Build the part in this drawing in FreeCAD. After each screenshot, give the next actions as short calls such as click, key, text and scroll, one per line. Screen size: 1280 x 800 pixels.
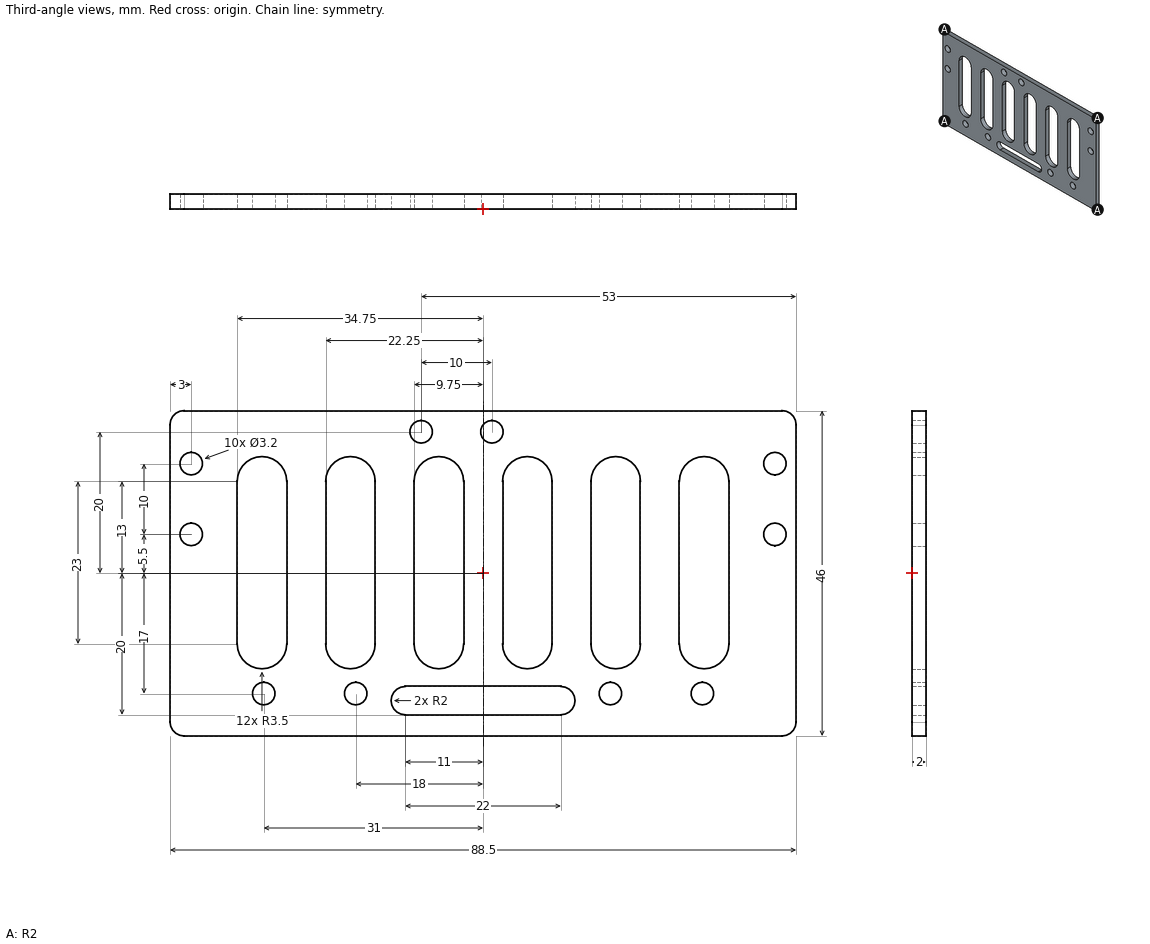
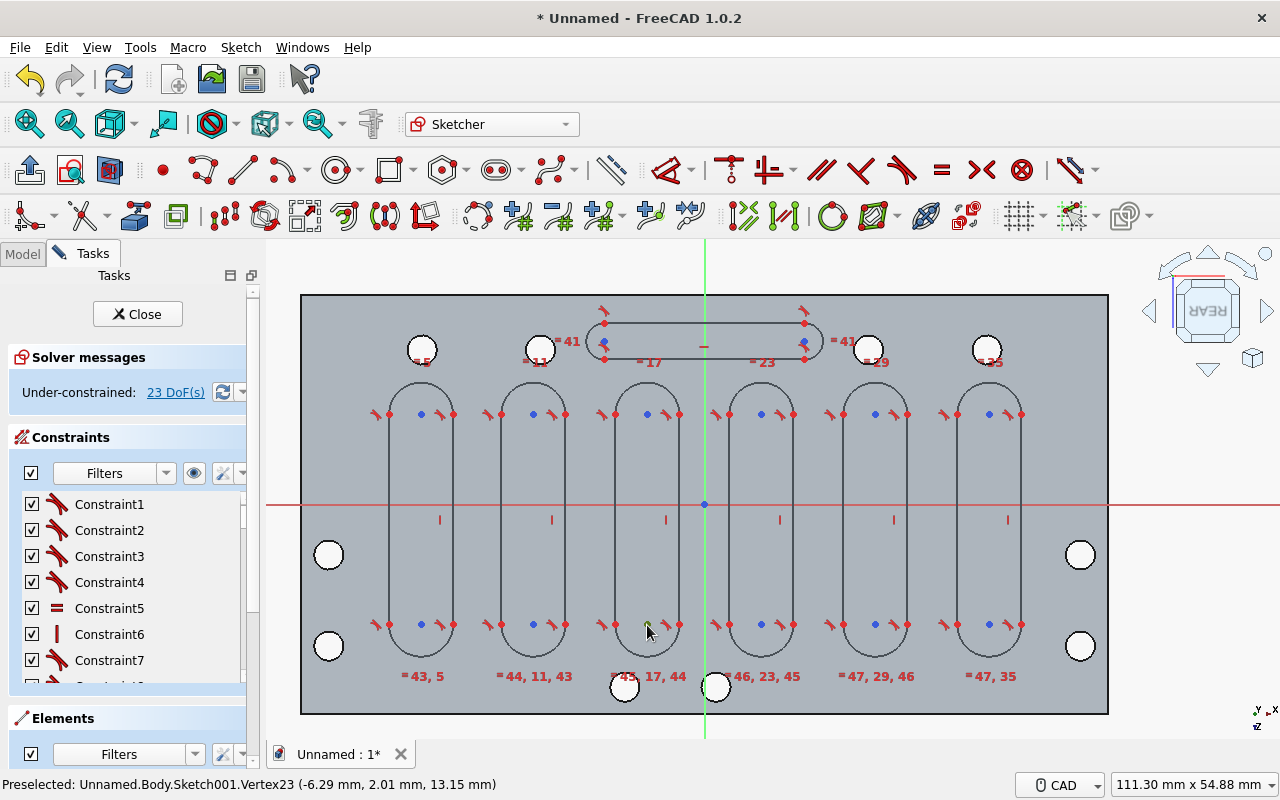
click(761, 625)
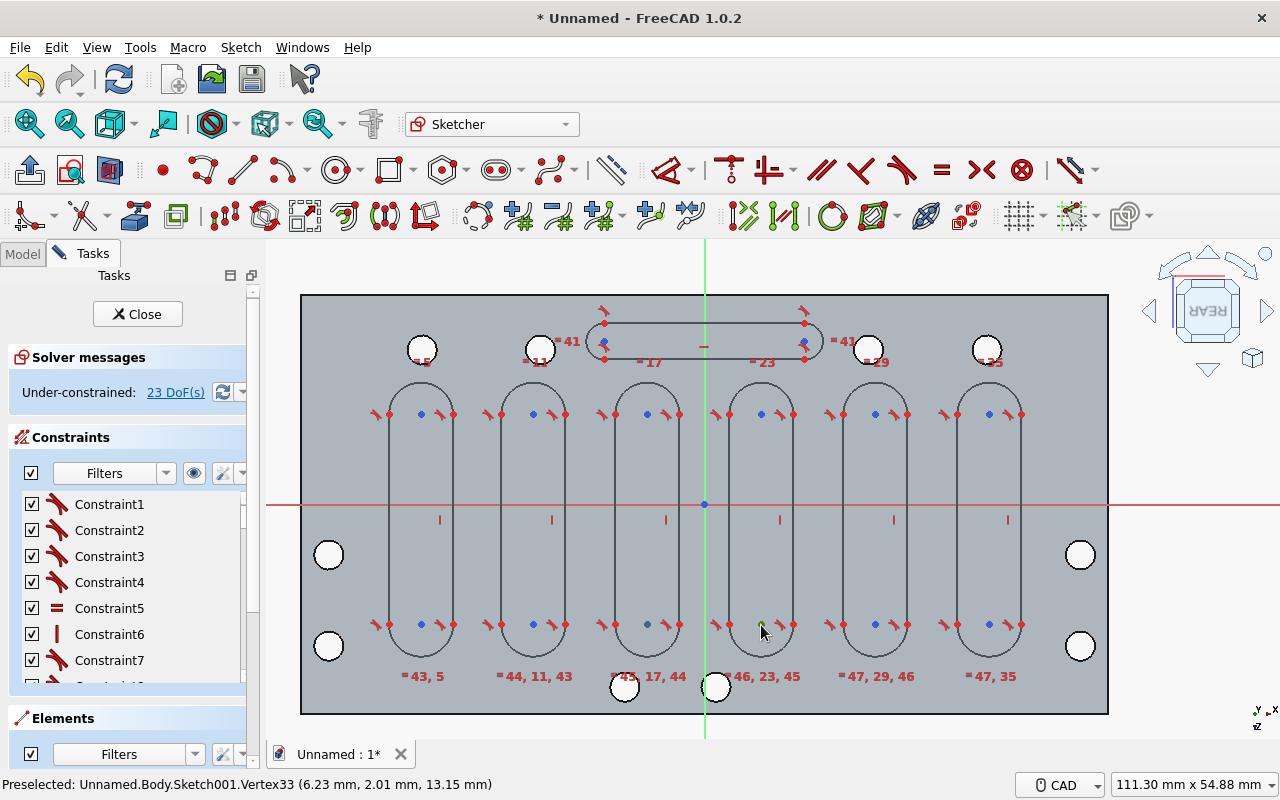
click(705, 679)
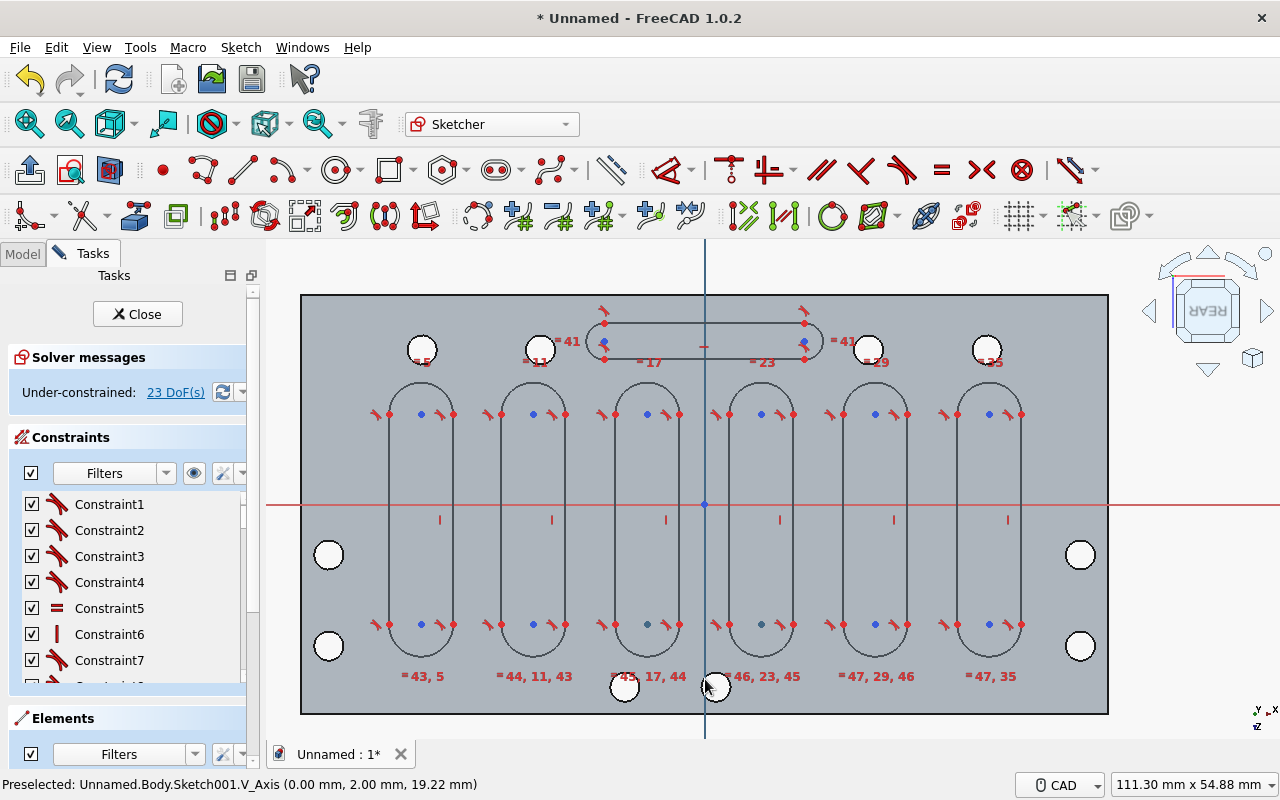
click(982, 170)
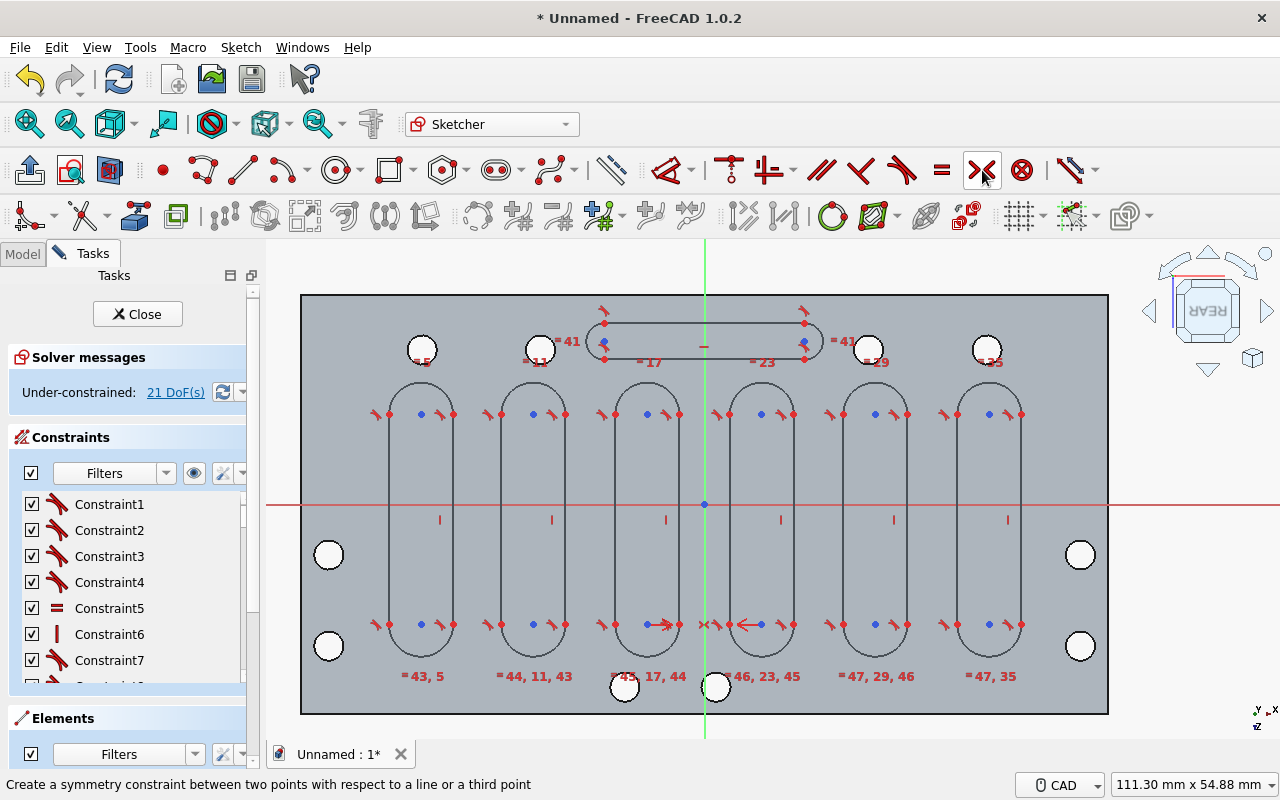
click(533, 625)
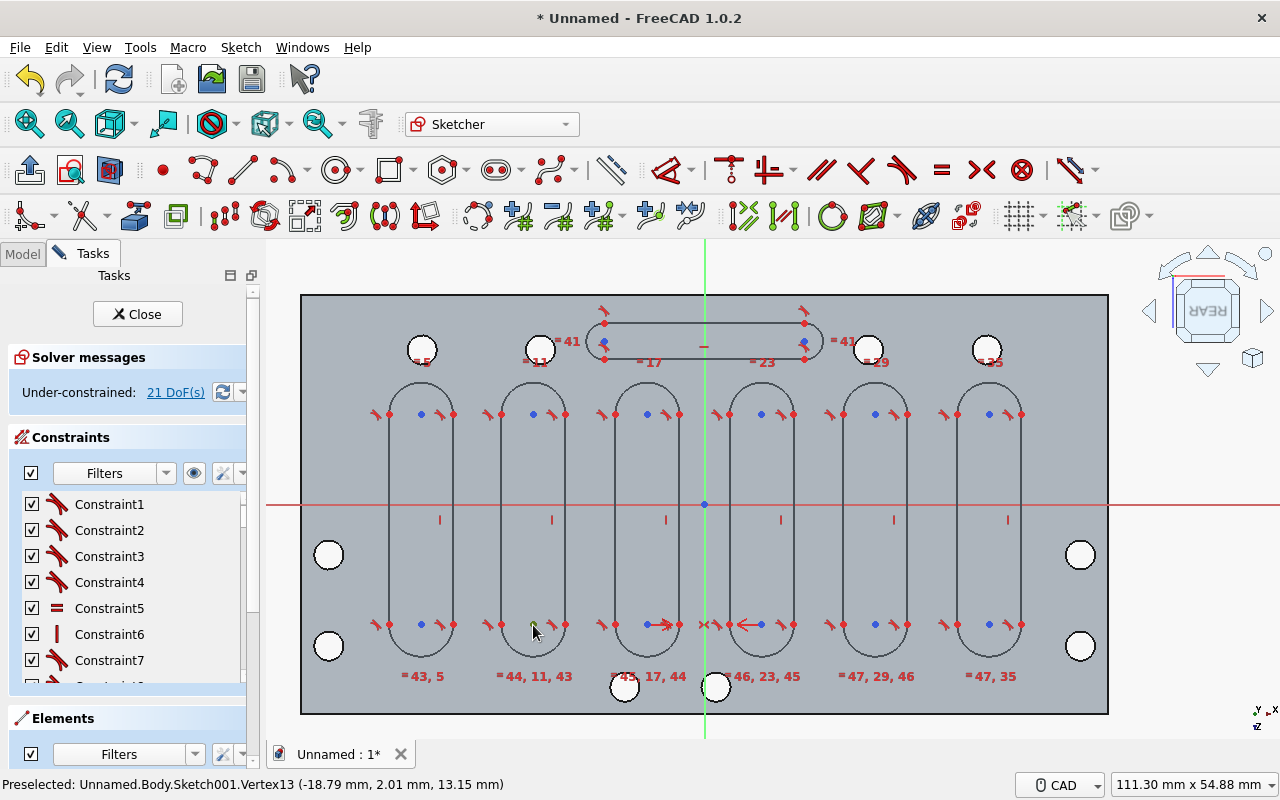
click(875, 625)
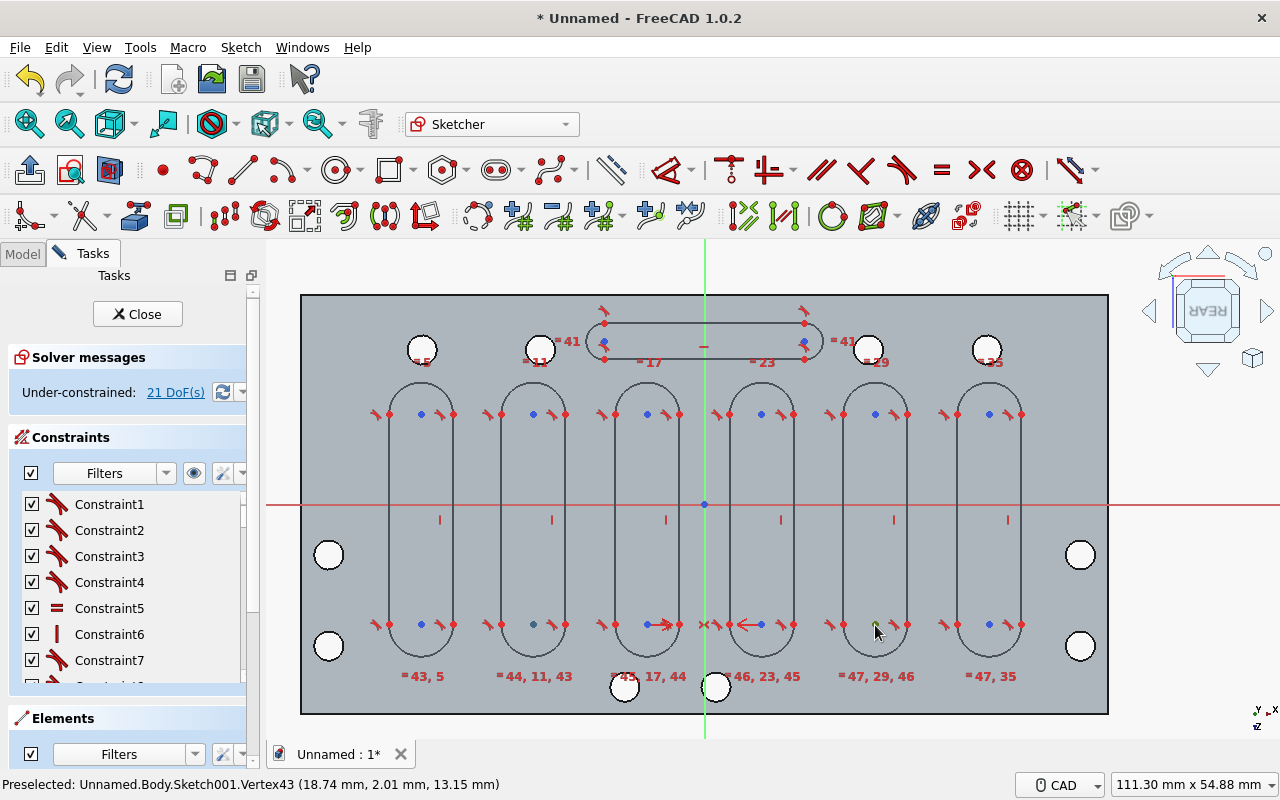
click(705, 679)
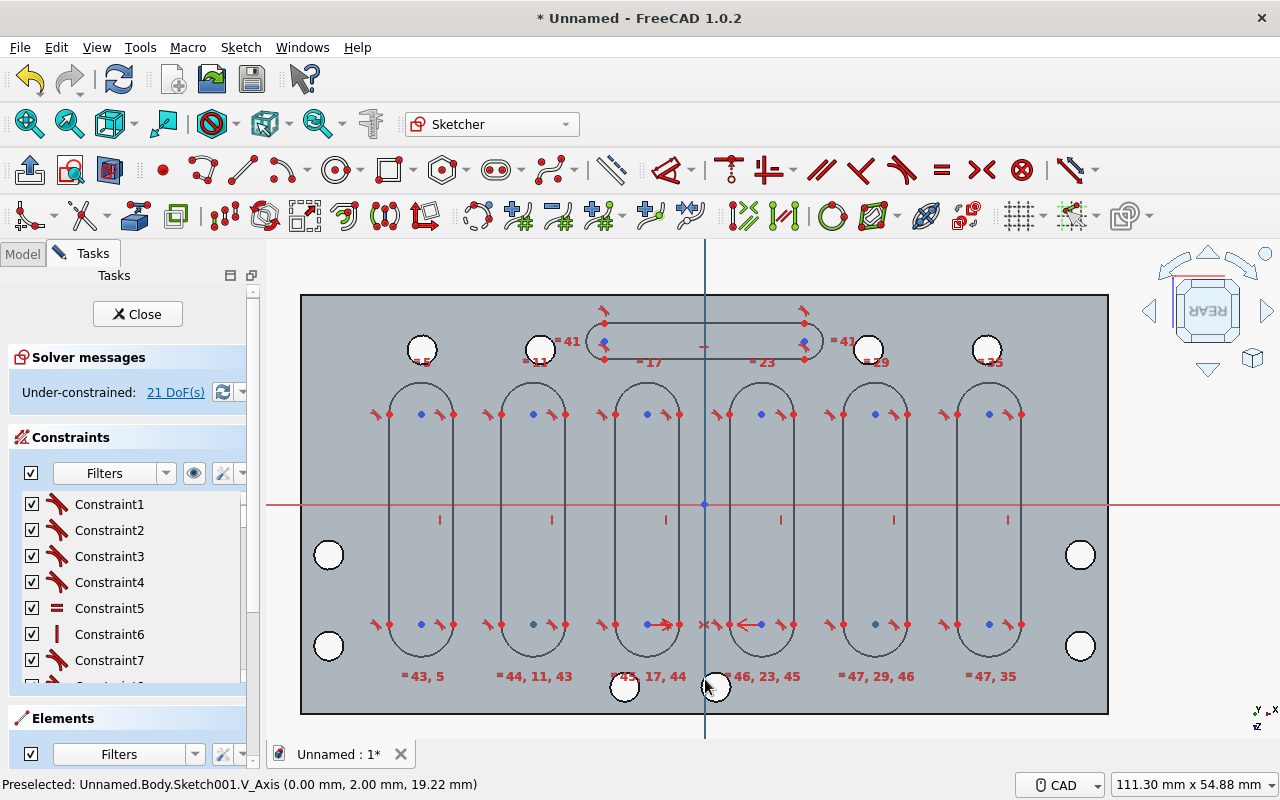
click(982, 170)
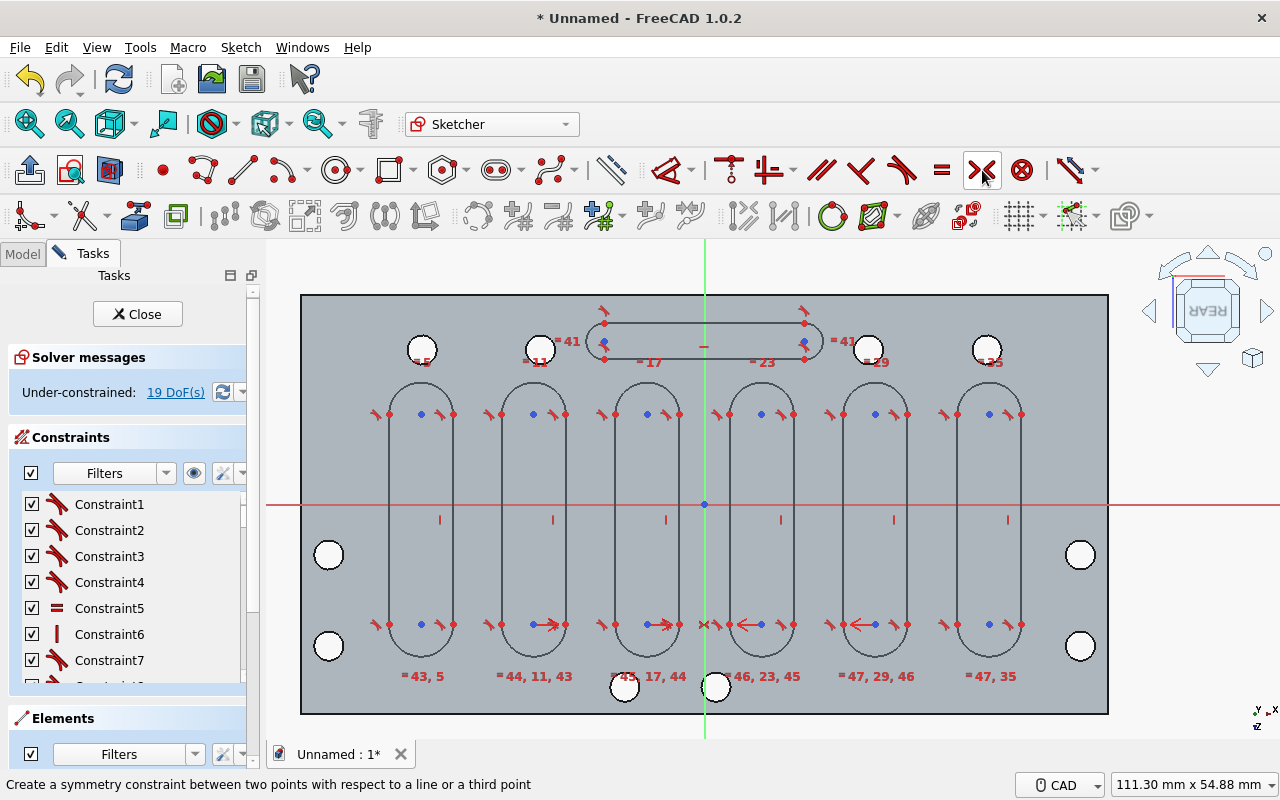
click(421, 625)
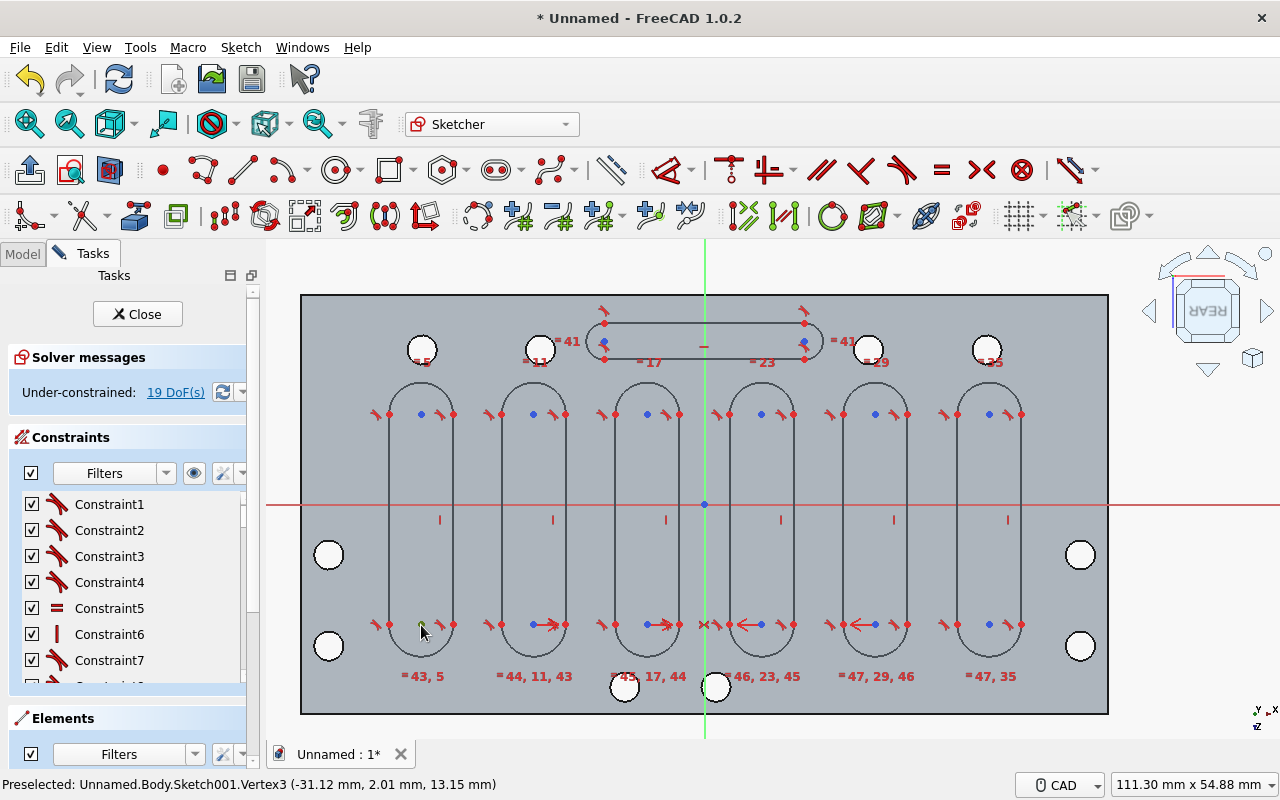
click(989, 625)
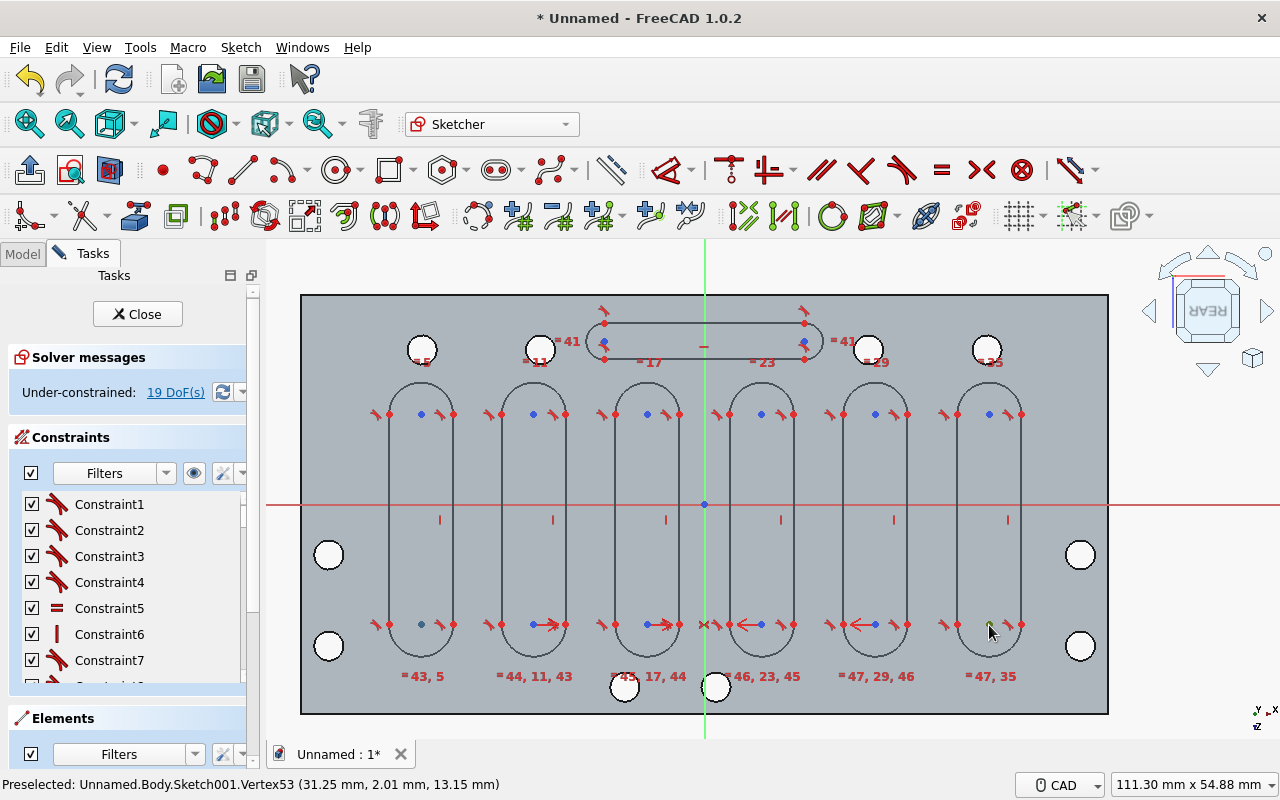
click(705, 679)